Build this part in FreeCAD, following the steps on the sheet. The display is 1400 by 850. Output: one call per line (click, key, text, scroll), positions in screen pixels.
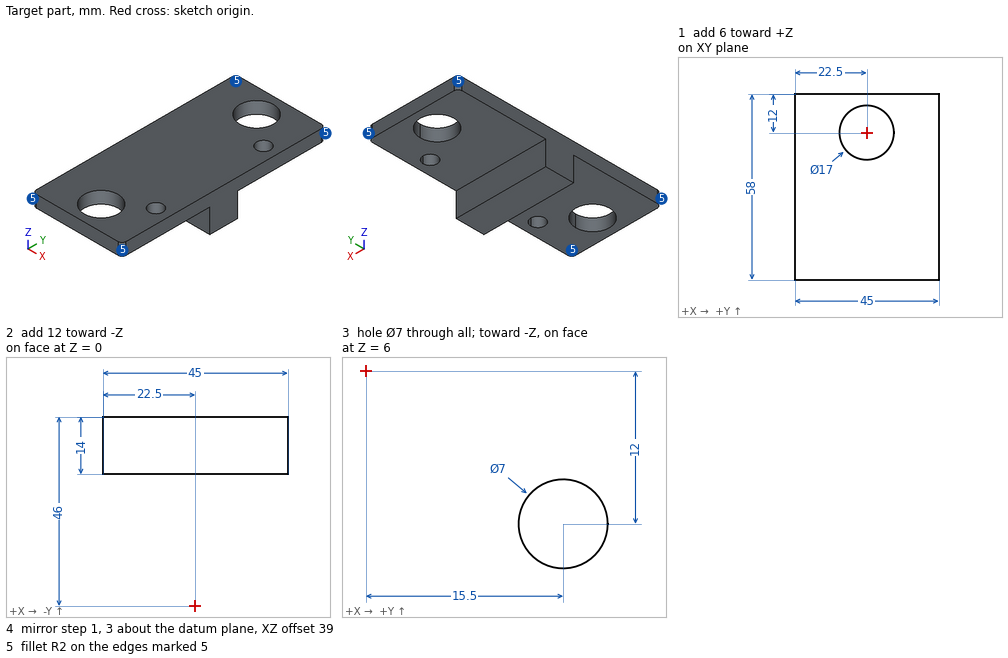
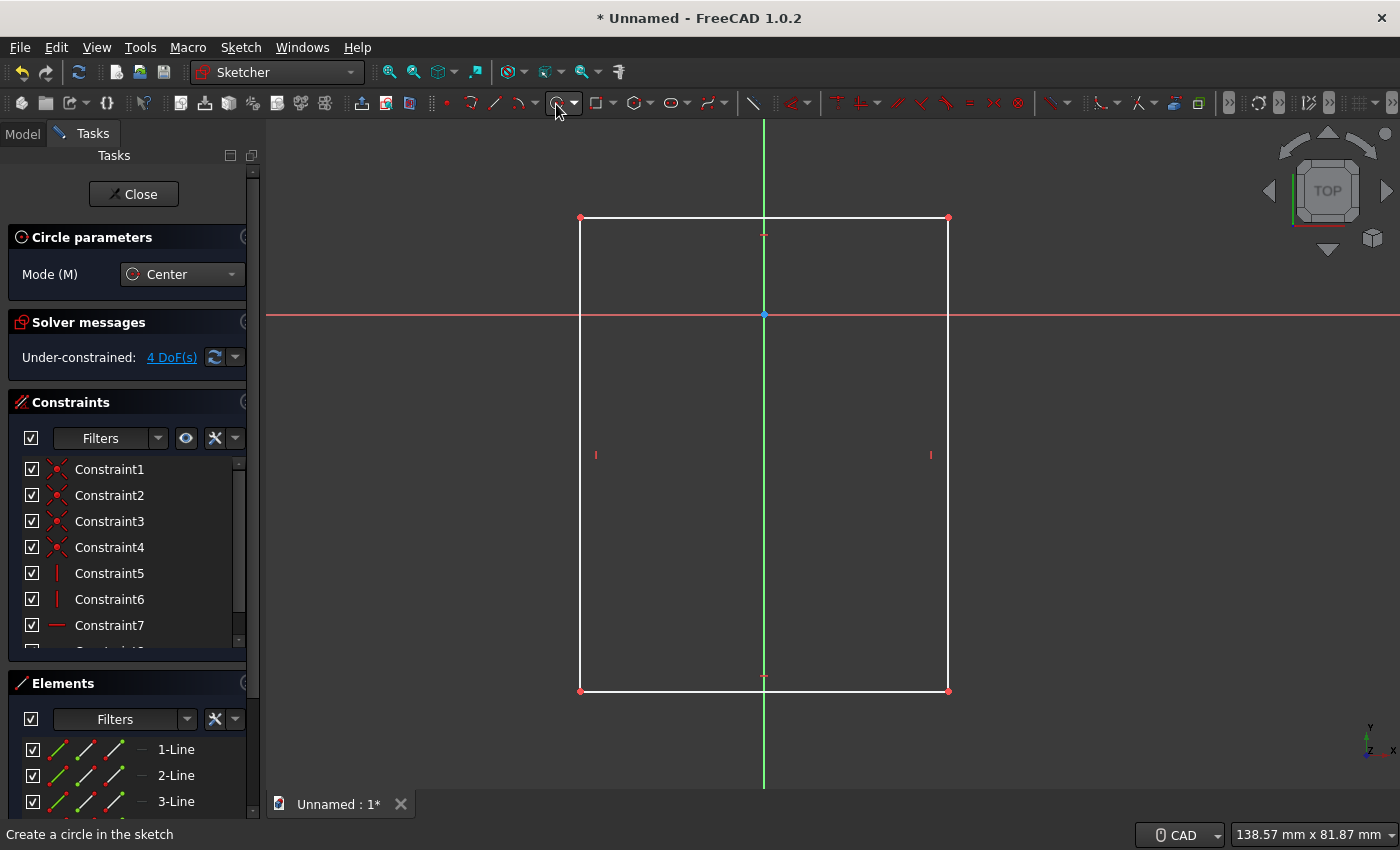
click(764, 315)
click(813, 266)
key(Escape)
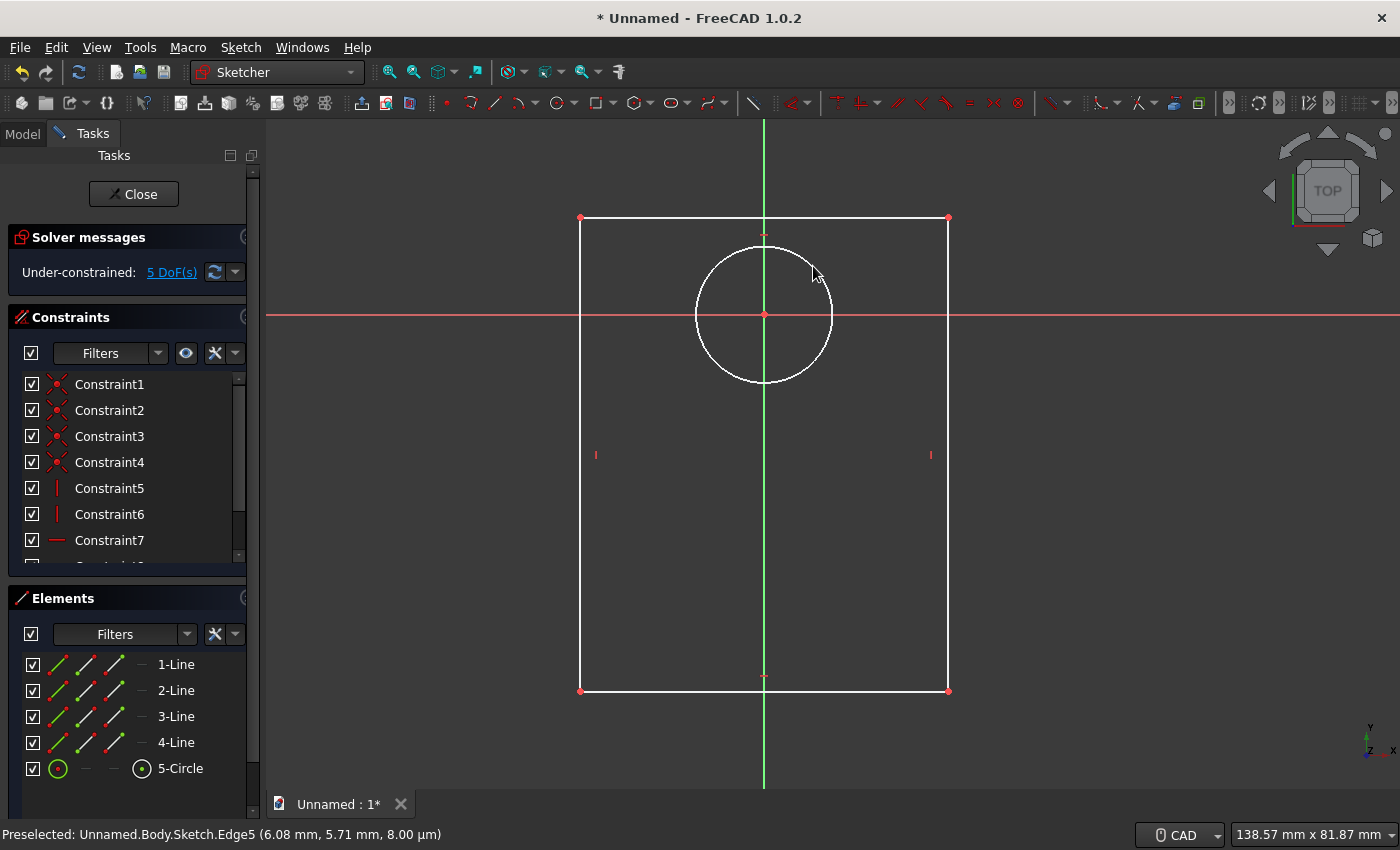
click(792, 104)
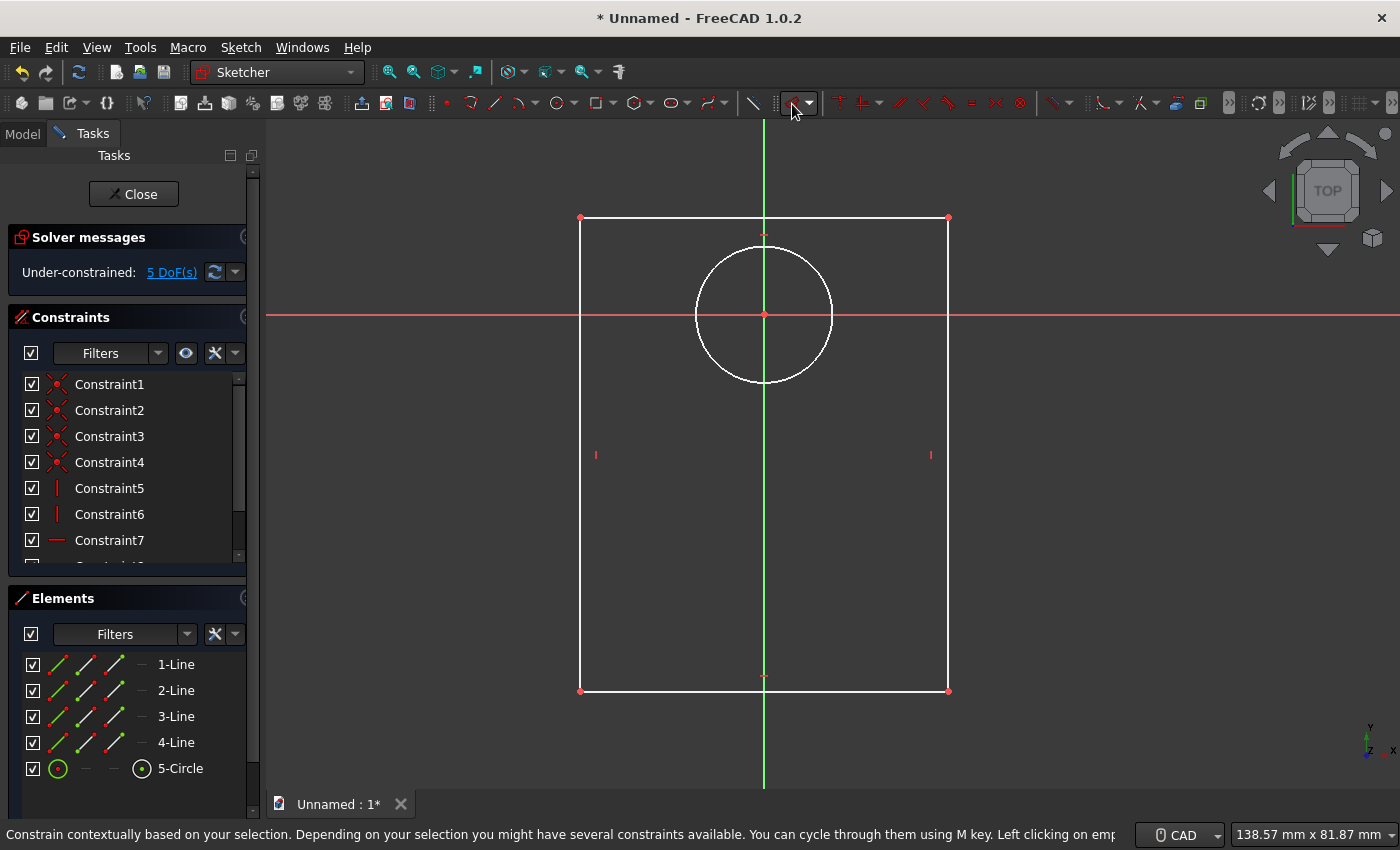
click(812, 266)
click(834, 243)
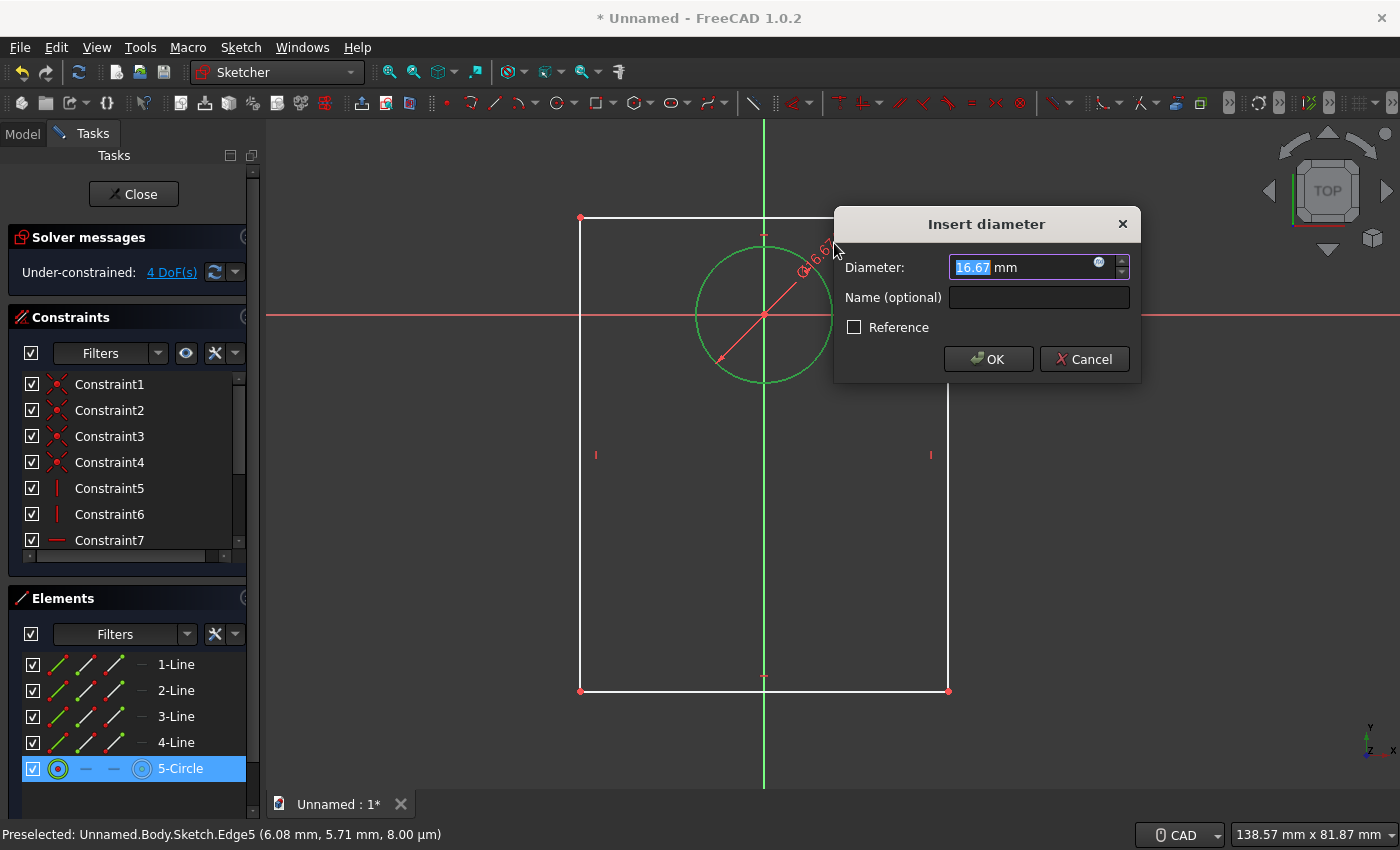
text(17)
key(Return)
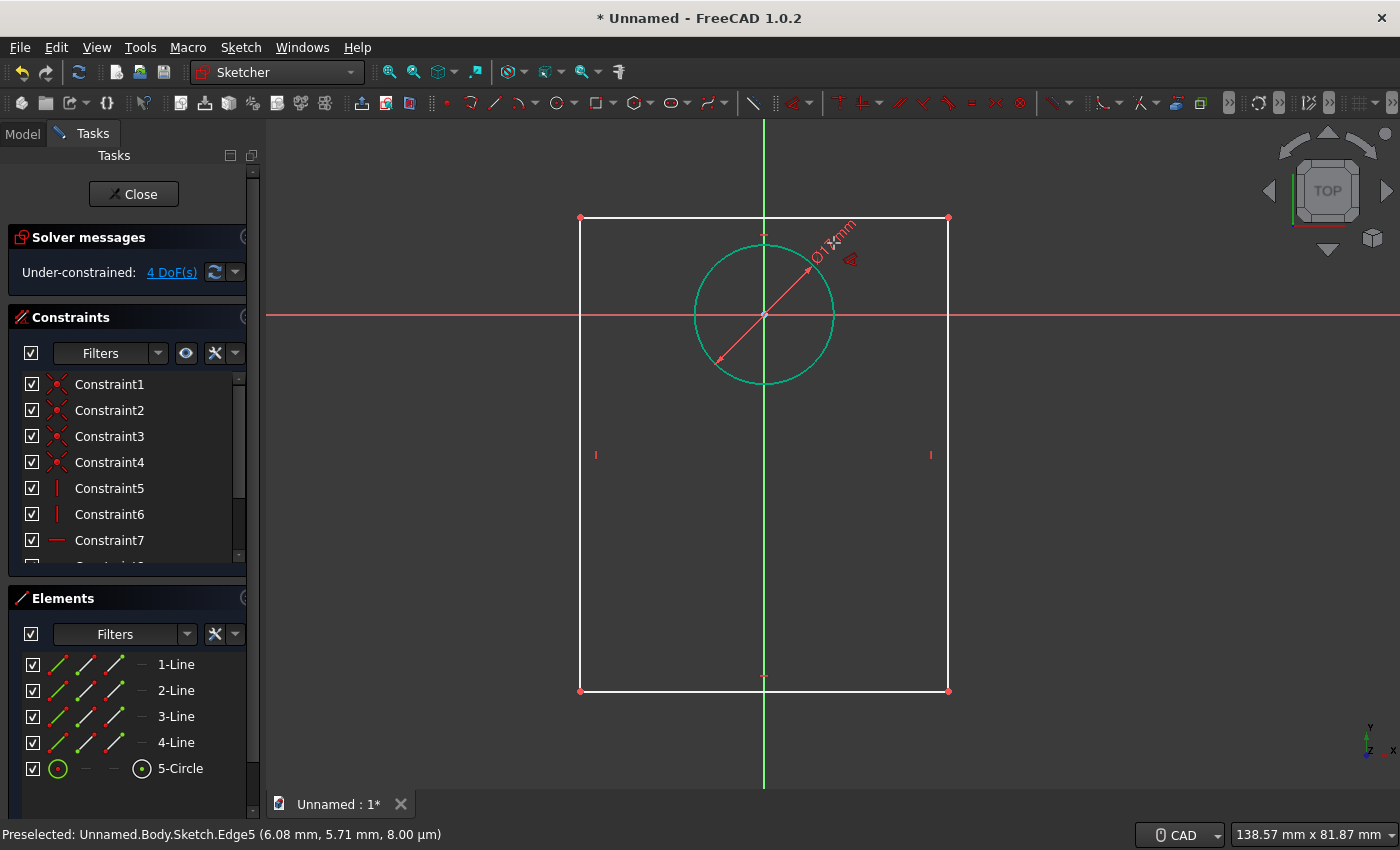
click(580, 360)
click(546, 455)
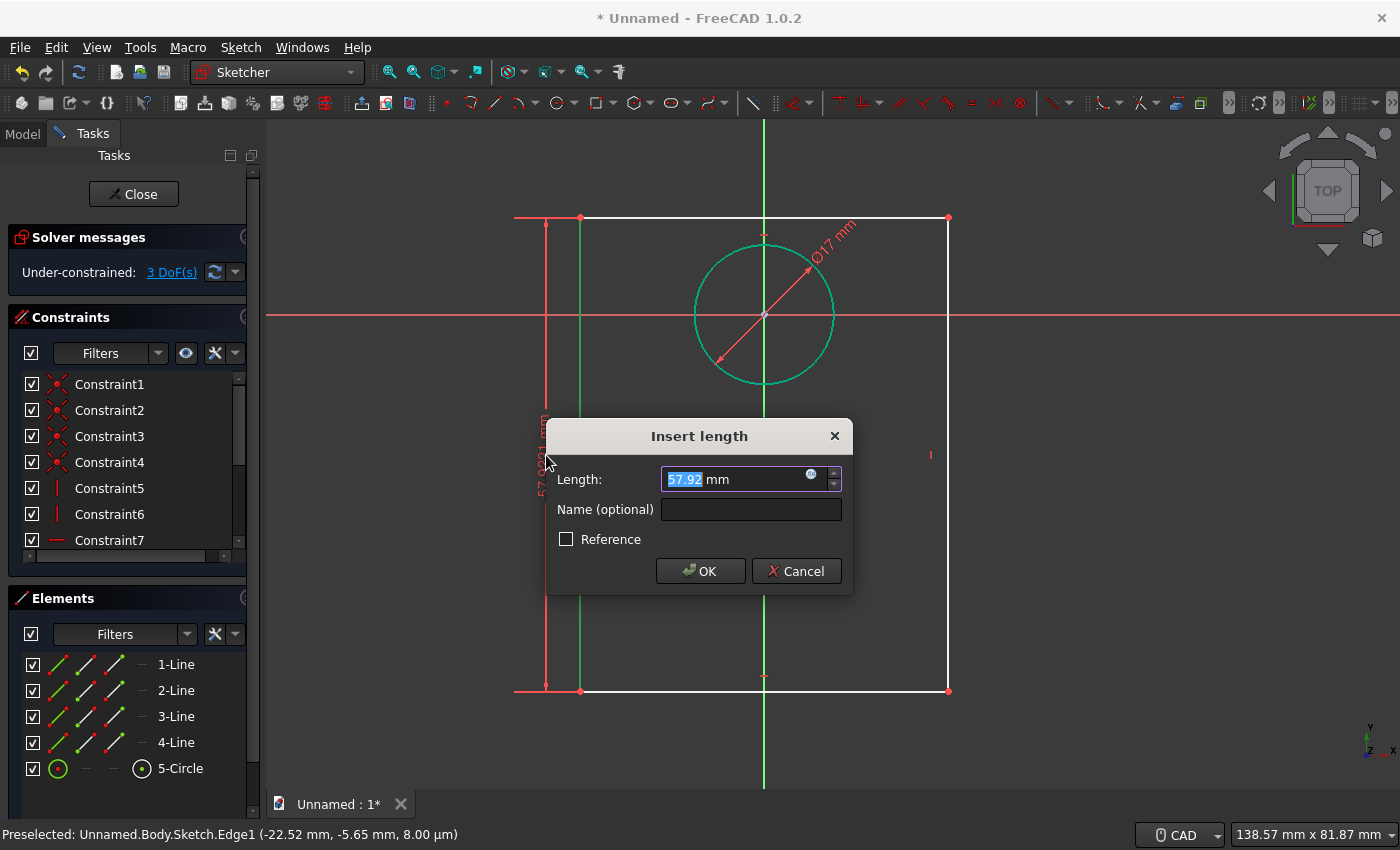
text(58)
key(Return)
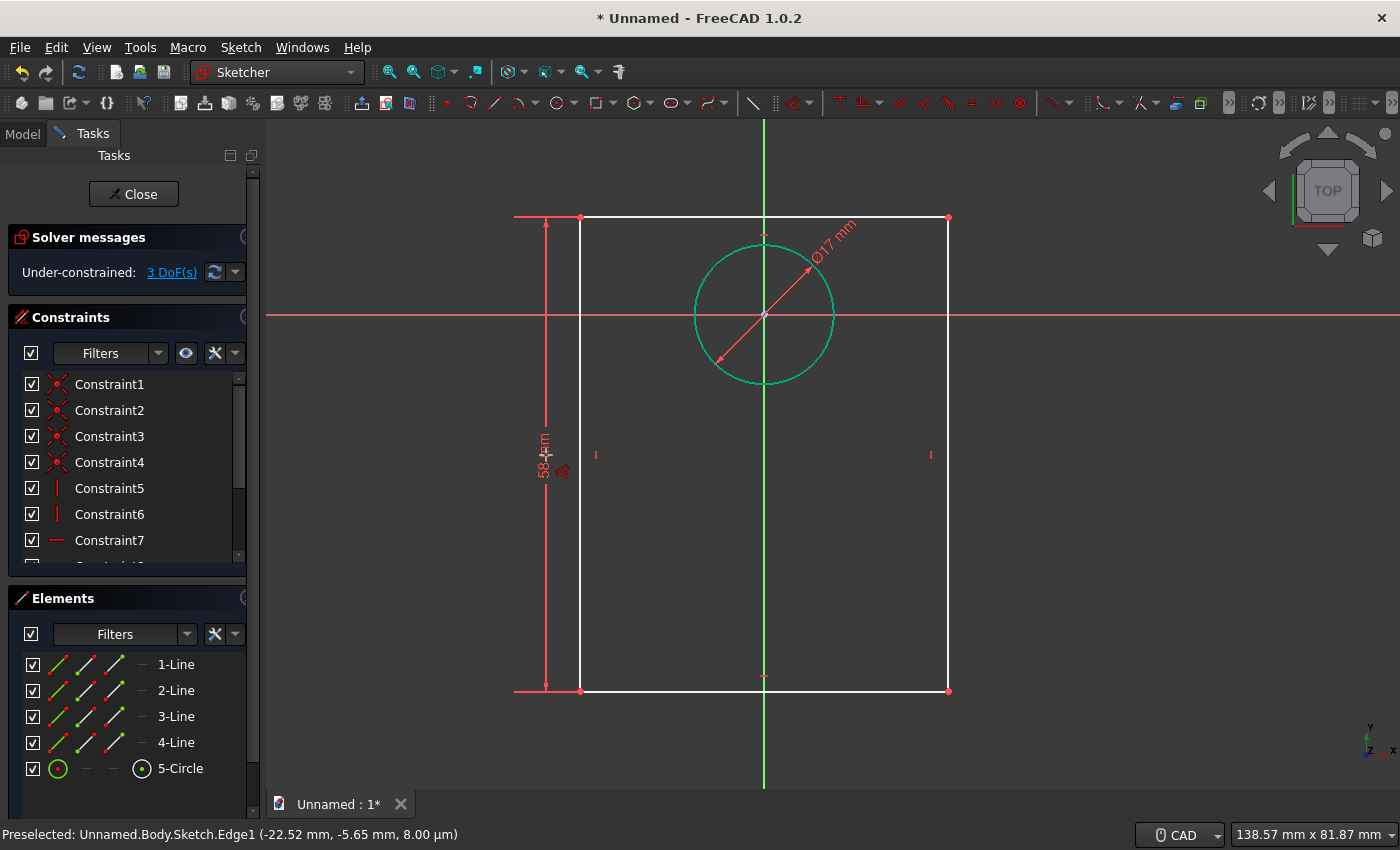
click(690, 692)
click(679, 726)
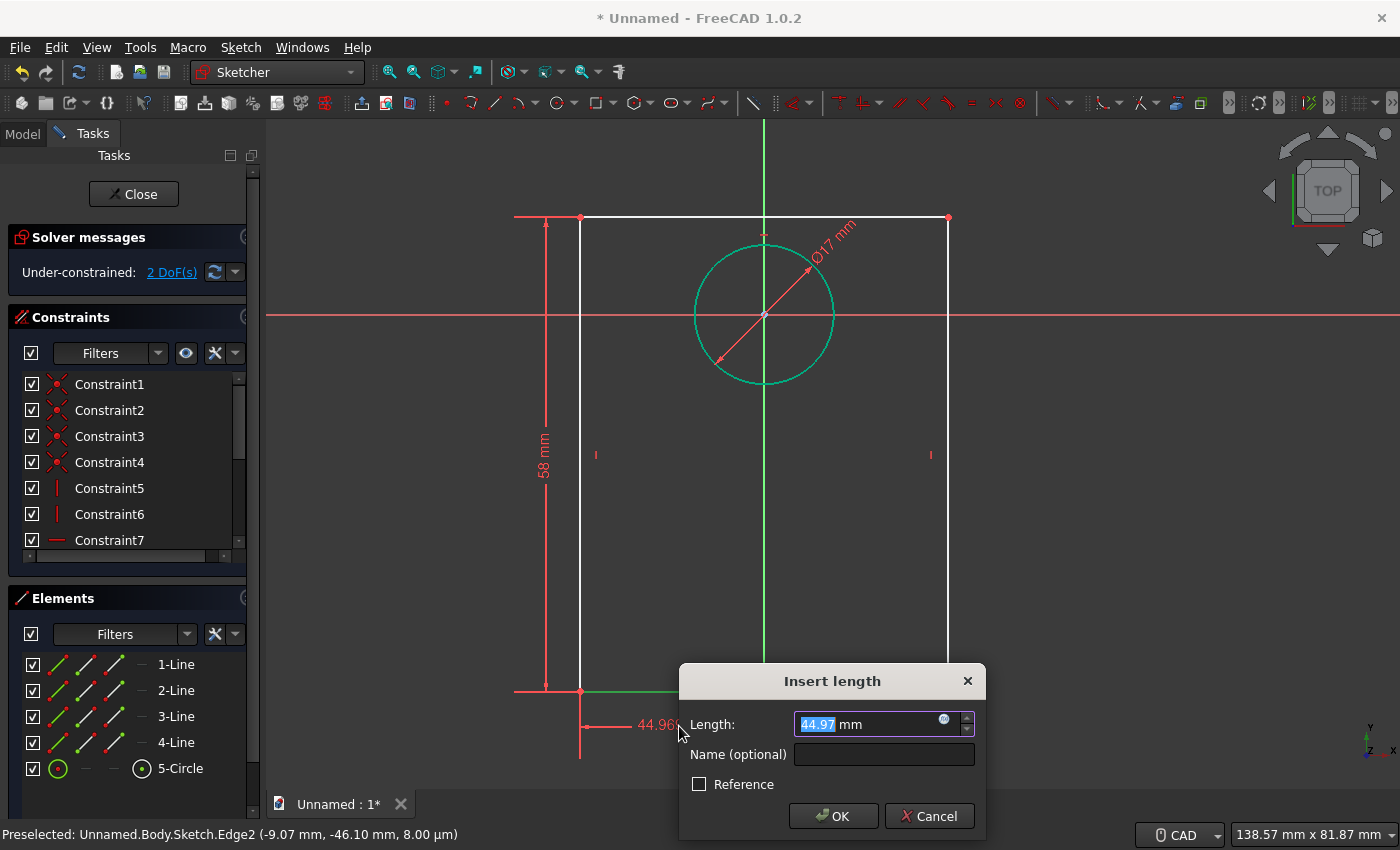
text(45)
key(Return)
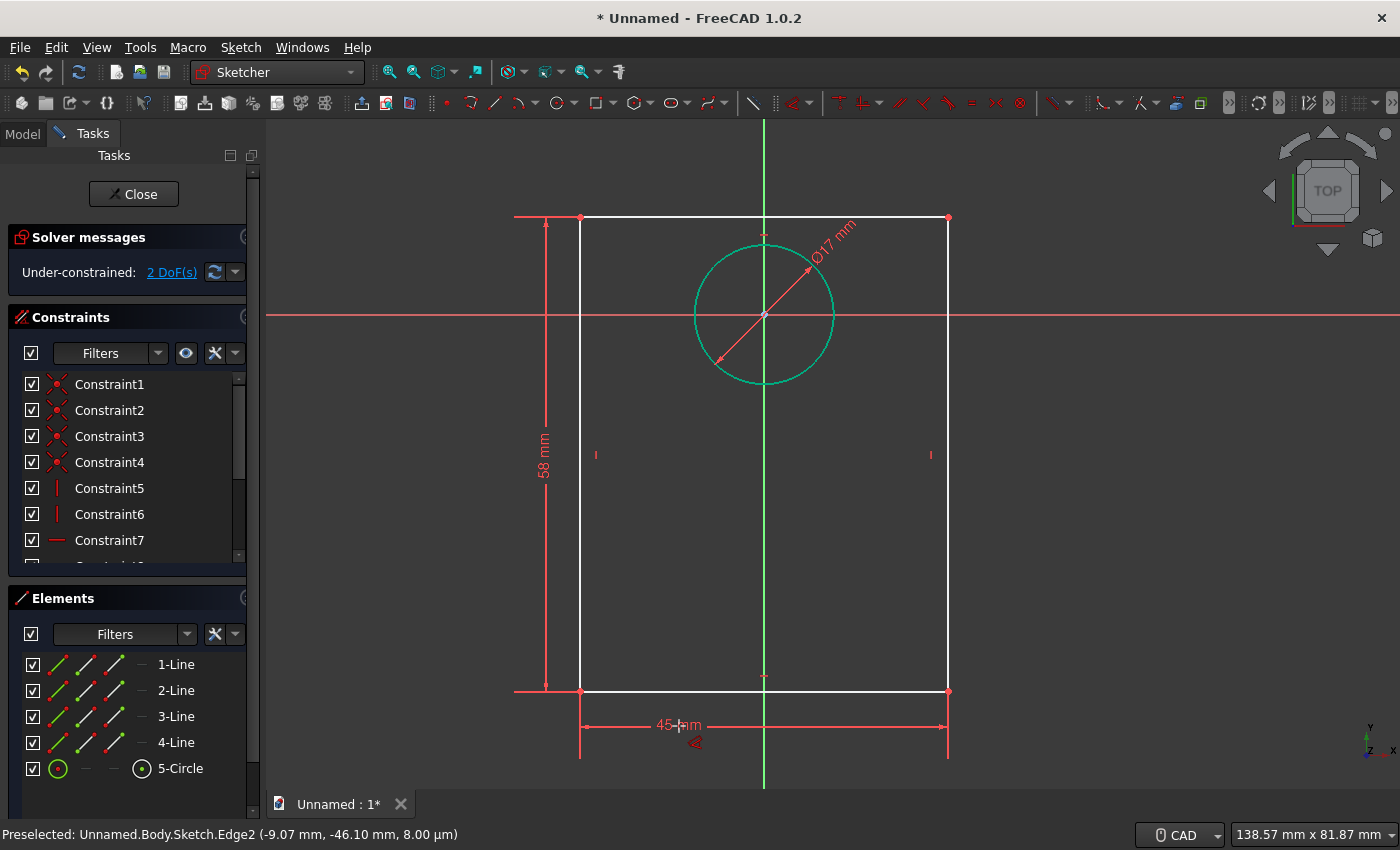
click(580, 217)
click(546, 266)